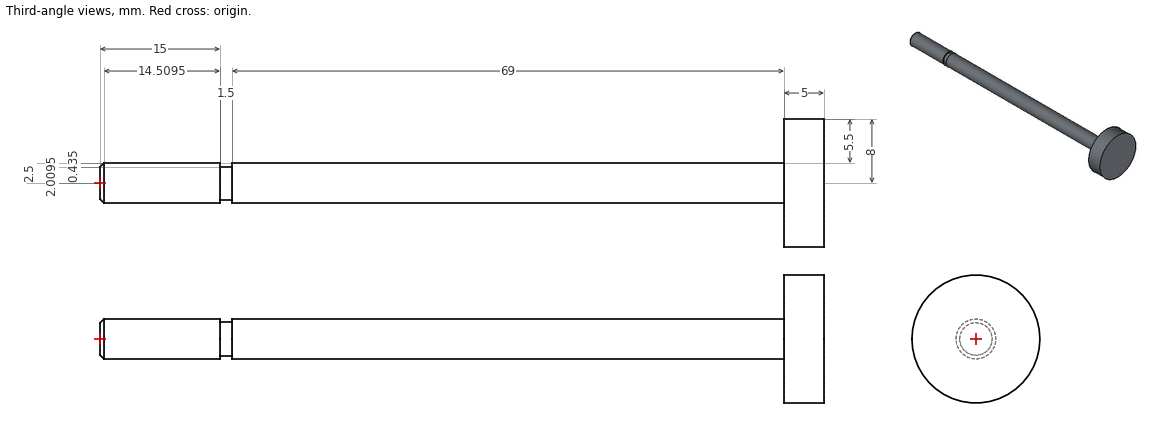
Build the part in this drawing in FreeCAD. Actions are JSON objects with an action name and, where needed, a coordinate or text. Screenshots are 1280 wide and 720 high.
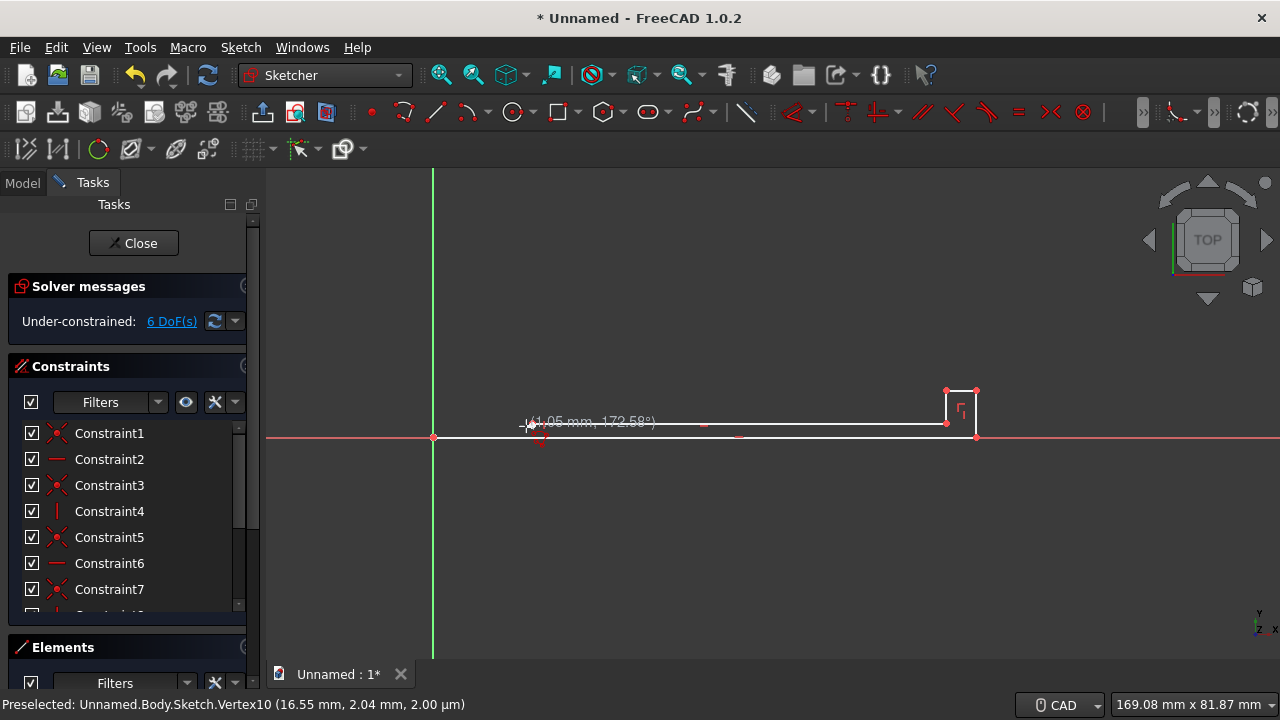
{"action": "scroll", "coordinate": [523, 426], "scroll_direction": "up", "scroll_amount": 3}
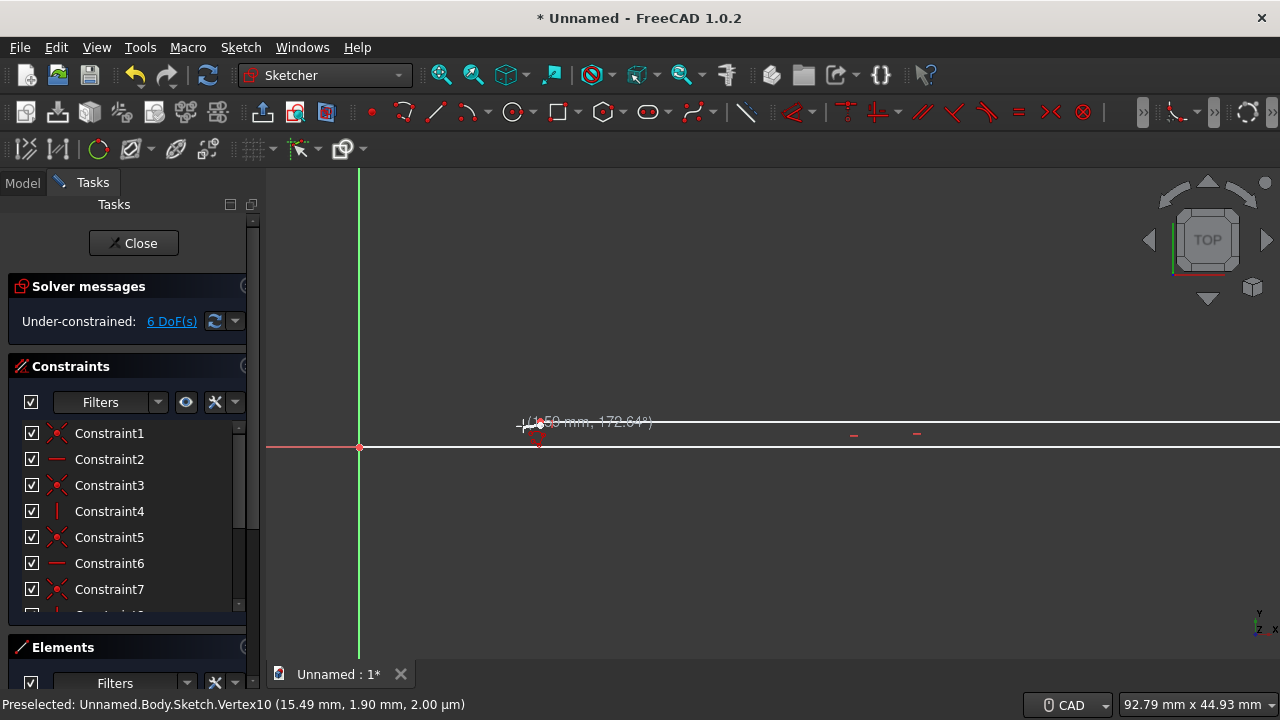
{"action": "left_click", "coordinate": [523, 425]}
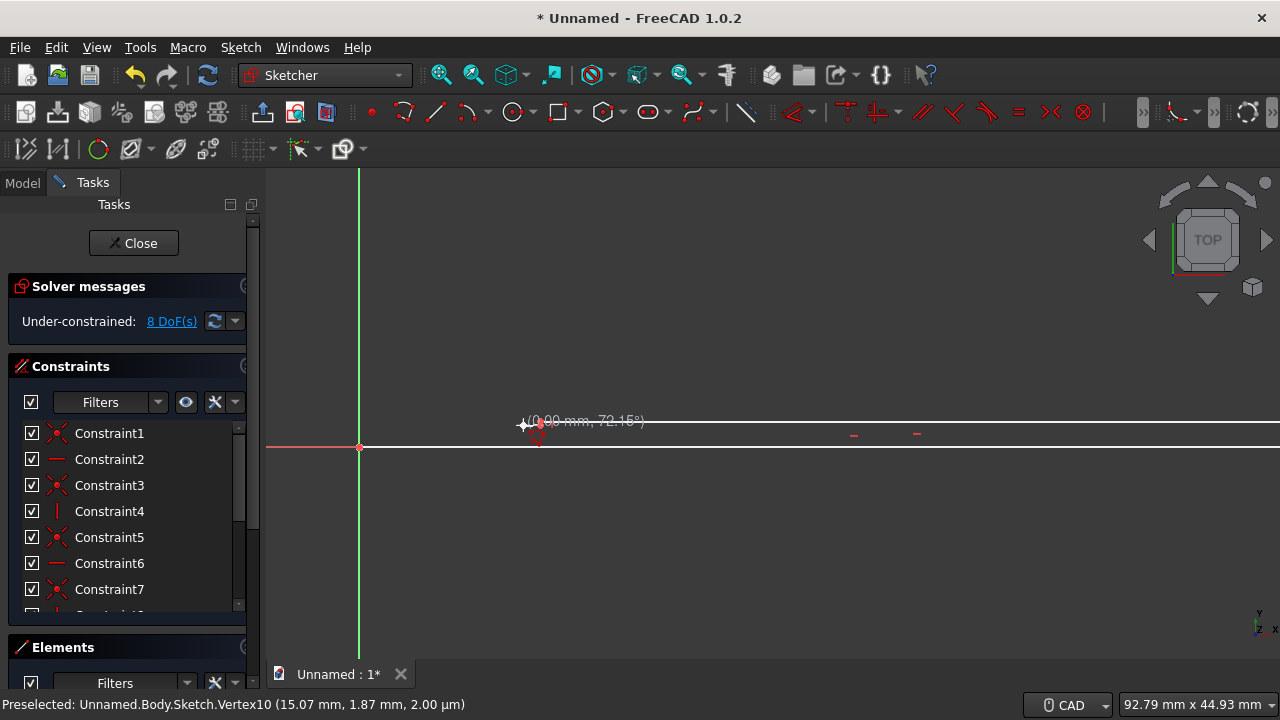
{"action": "scroll", "coordinate": [523, 420], "scroll_direction": "up", "scroll_amount": 7}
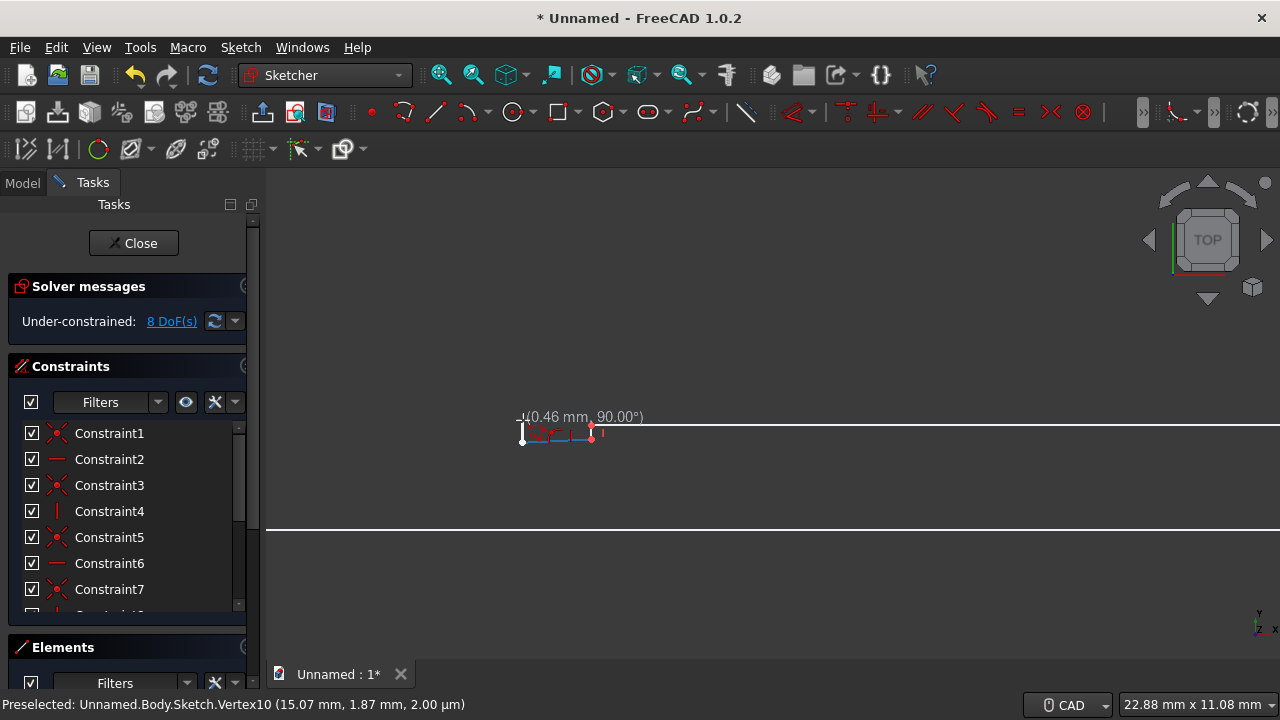
{"action": "left_click", "coordinate": [522, 419]}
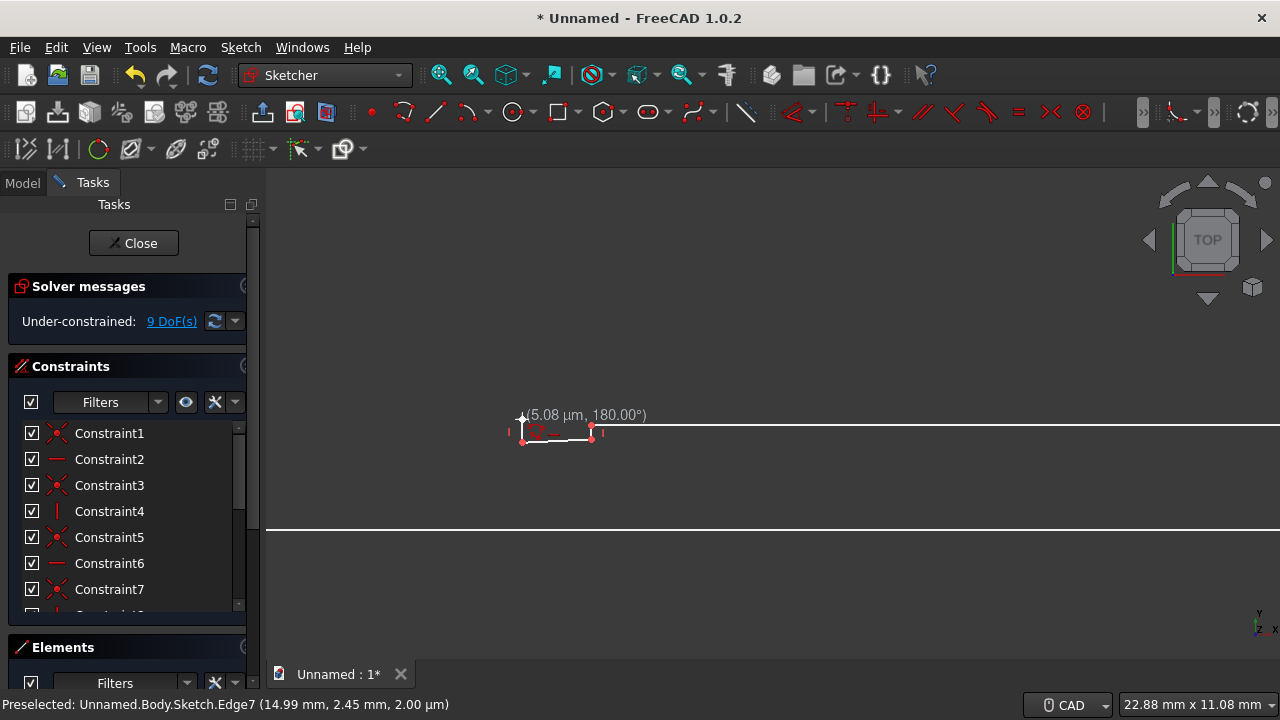
{"action": "scroll", "coordinate": [523, 423], "scroll_direction": "down", "scroll_amount": 10}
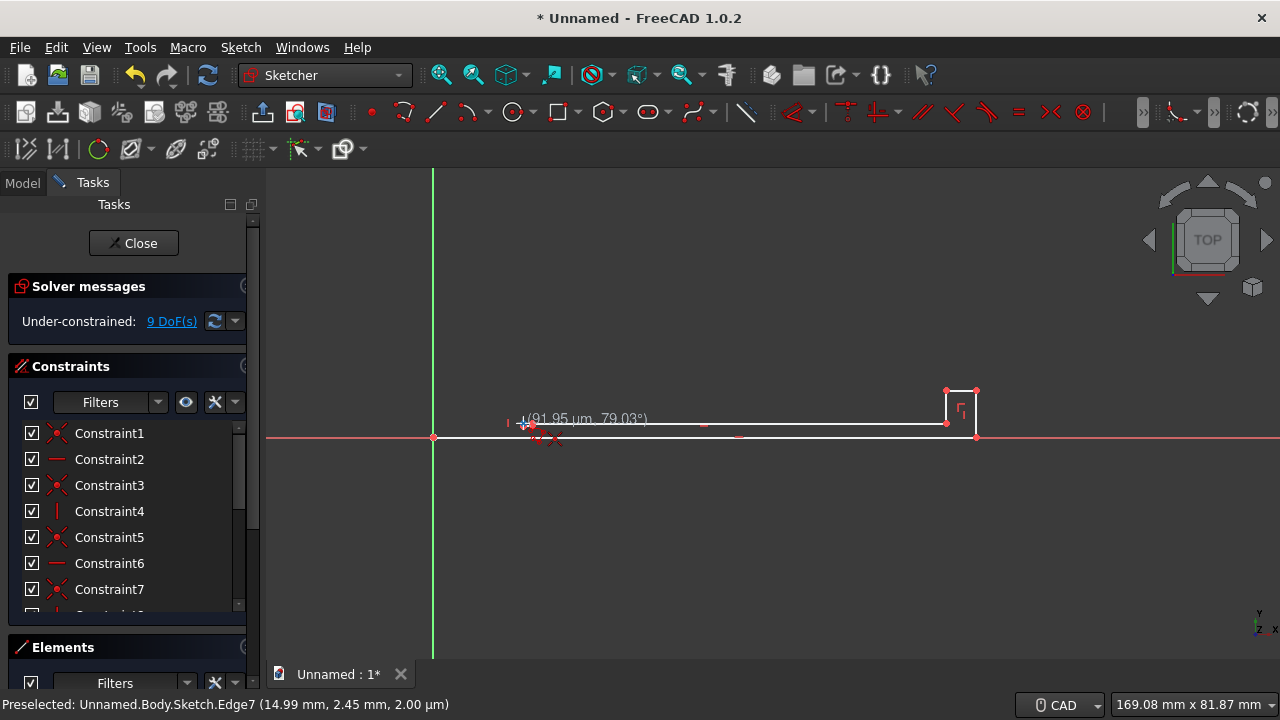
{"action": "scroll", "coordinate": [436, 423], "scroll_direction": "up", "scroll_amount": 9}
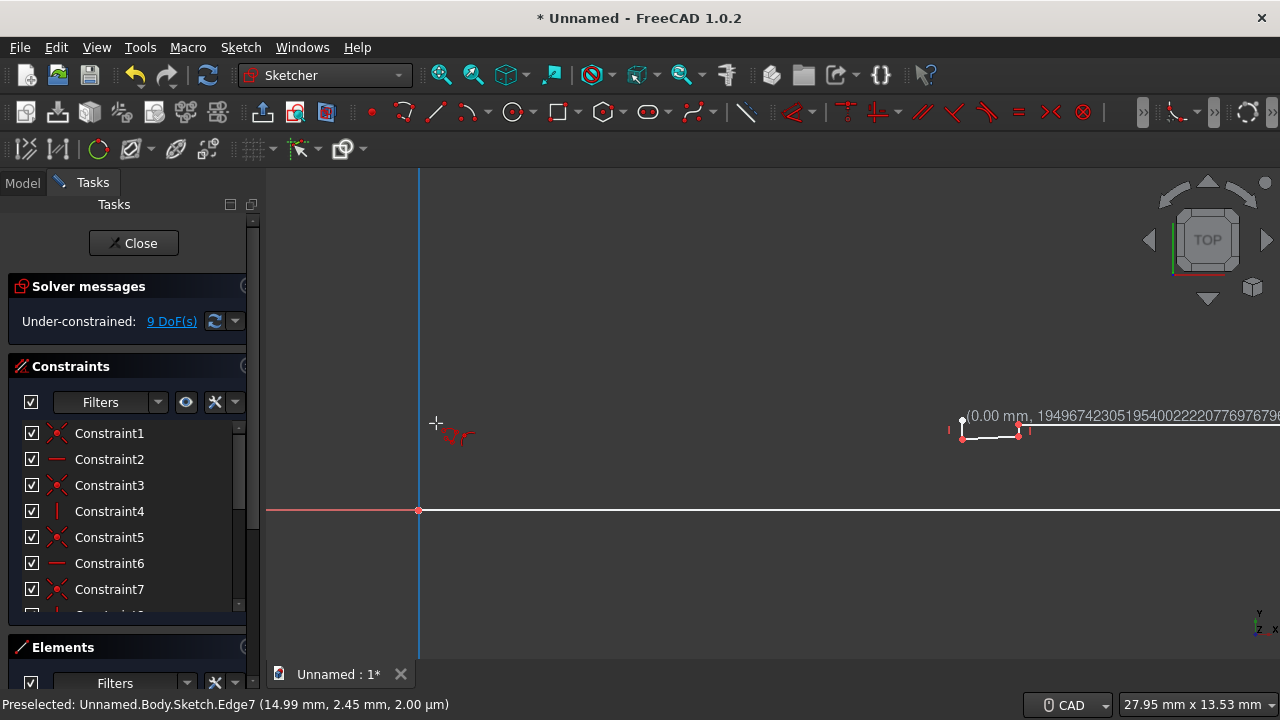
{"action": "left_click", "coordinate": [437, 420]}
{"action": "left_click", "coordinate": [428, 437]}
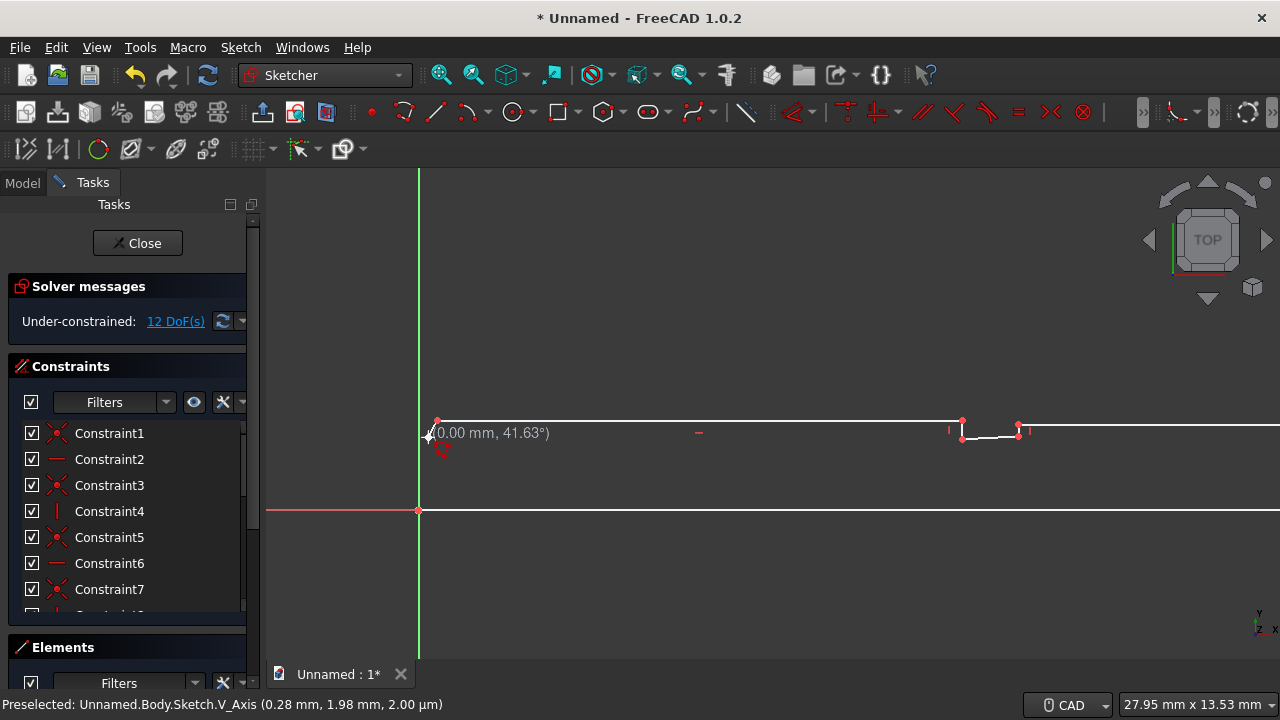
{"action": "scroll", "coordinate": [436, 423], "scroll_direction": "down", "scroll_amount": 9}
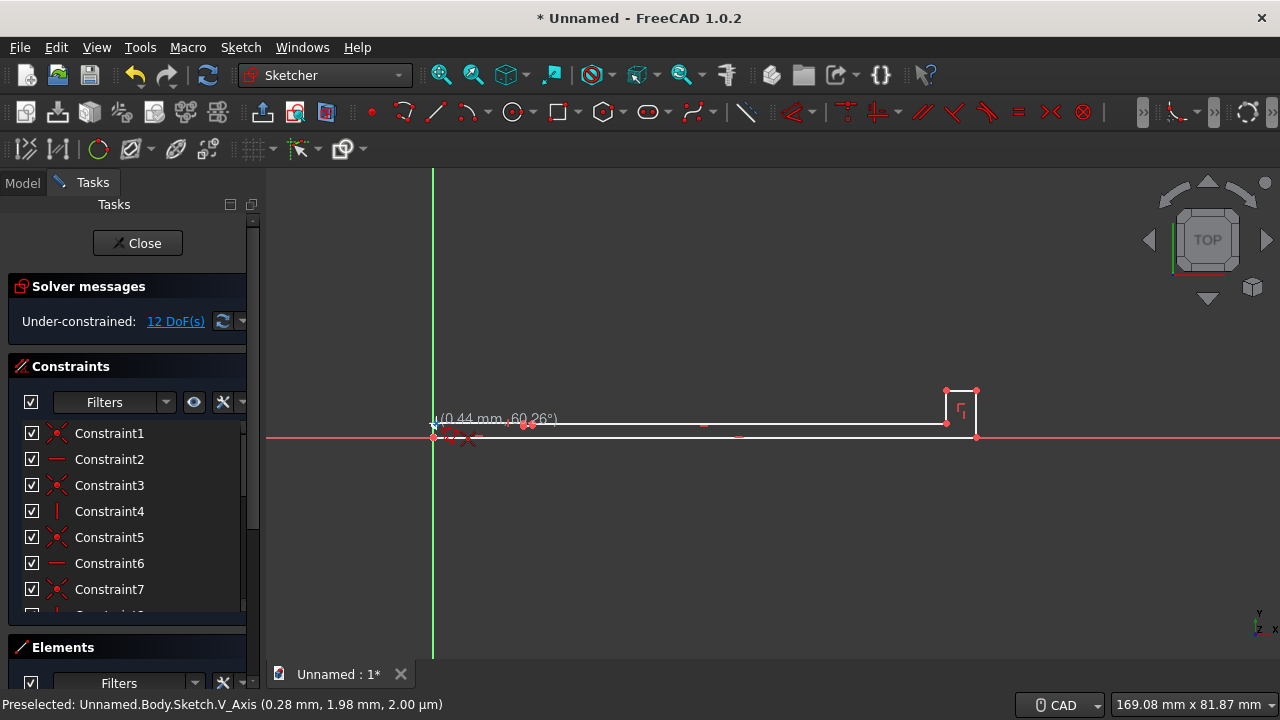
{"action": "scroll", "coordinate": [433, 438], "scroll_direction": "up", "scroll_amount": 2}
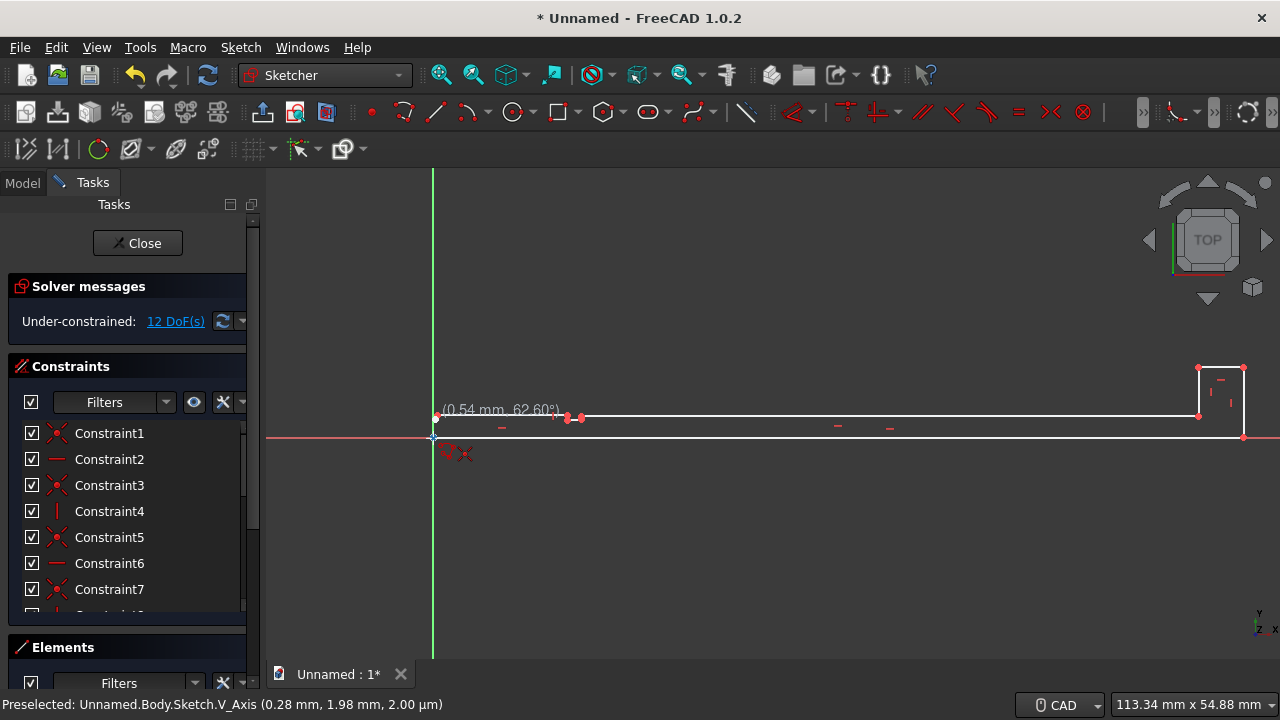
{"action": "left_click", "coordinate": [433, 438]}
{"action": "key", "text": "Escape"}
{"action": "key", "text": "Escape"}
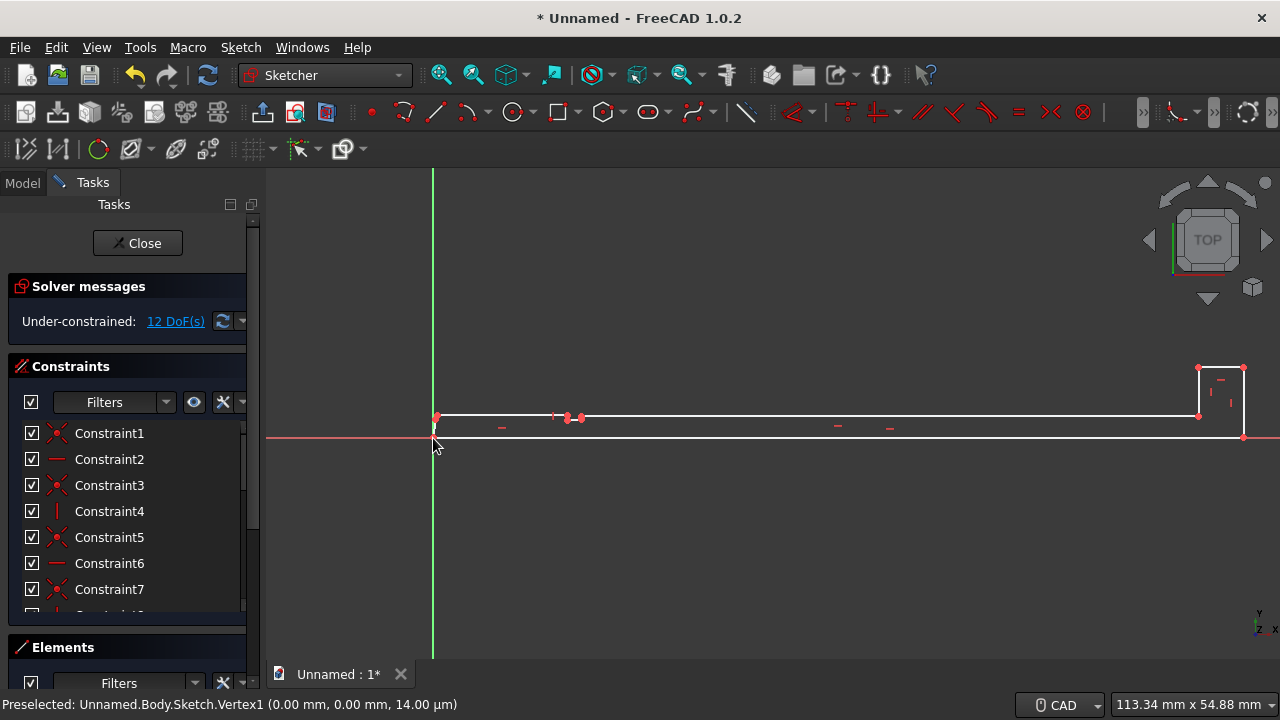
{"action": "scroll", "coordinate": [574, 420], "scroll_direction": "up", "scroll_amount": 4}